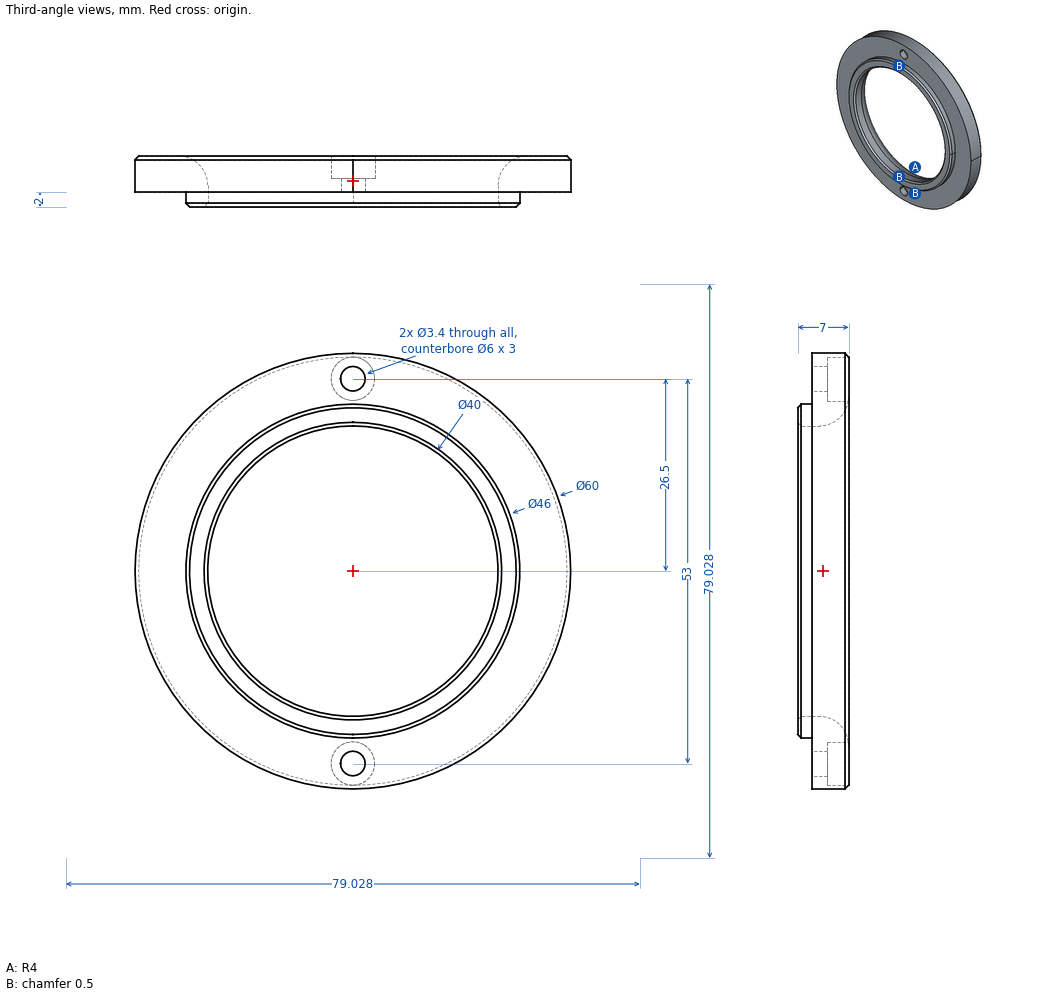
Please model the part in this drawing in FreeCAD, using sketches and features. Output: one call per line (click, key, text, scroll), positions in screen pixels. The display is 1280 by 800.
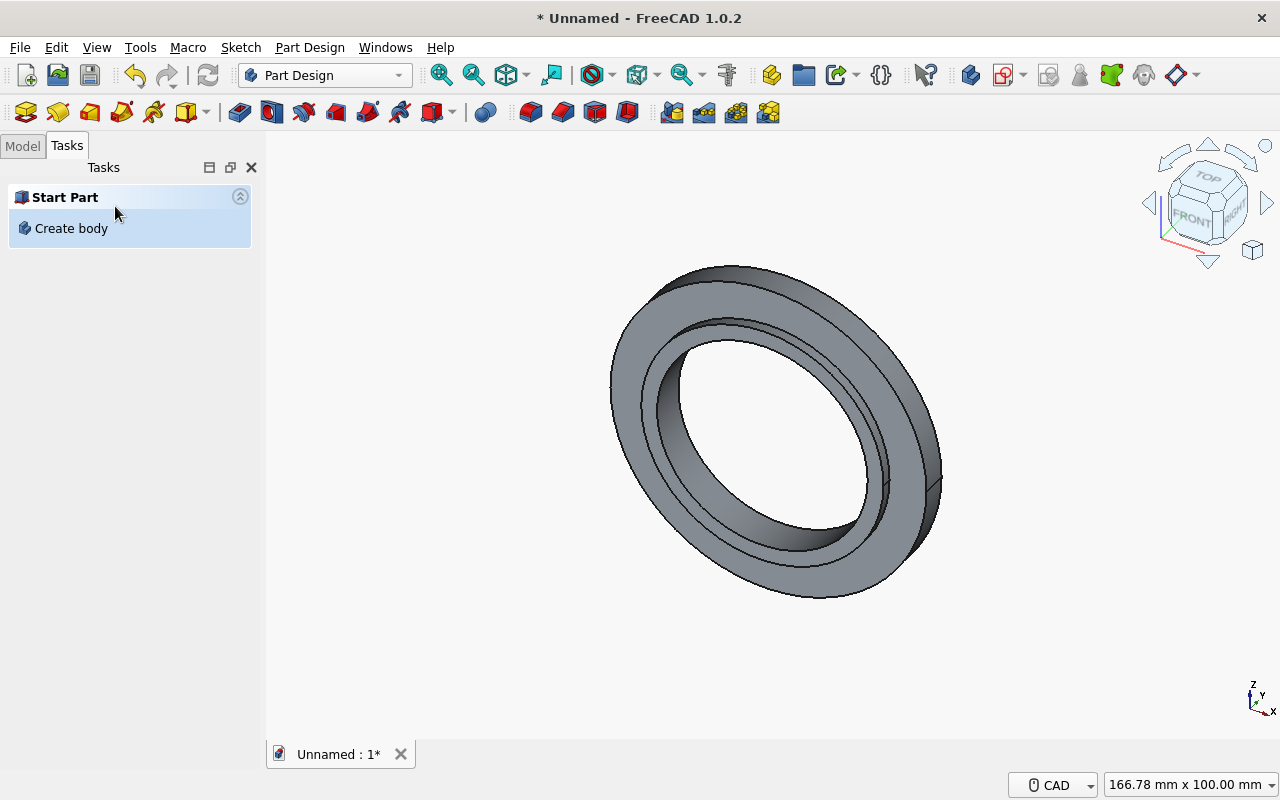
key(0)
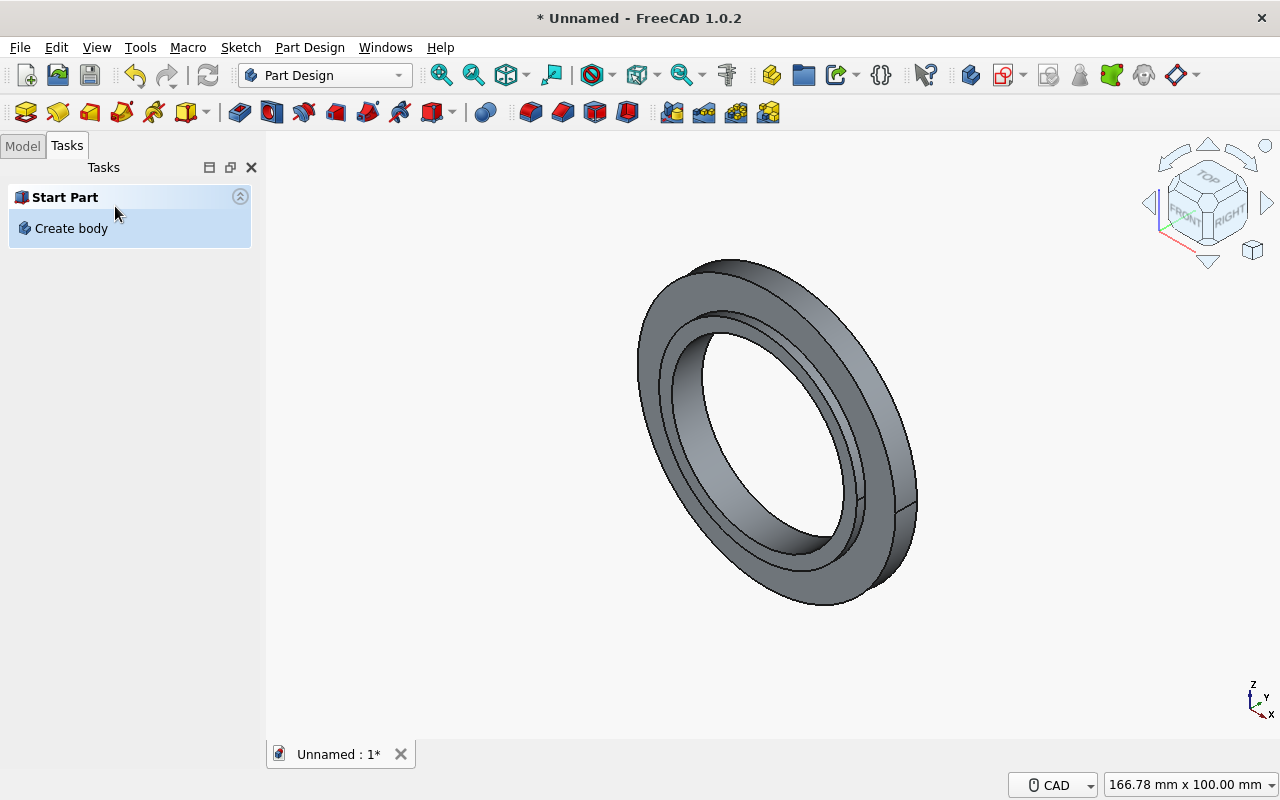
key(2)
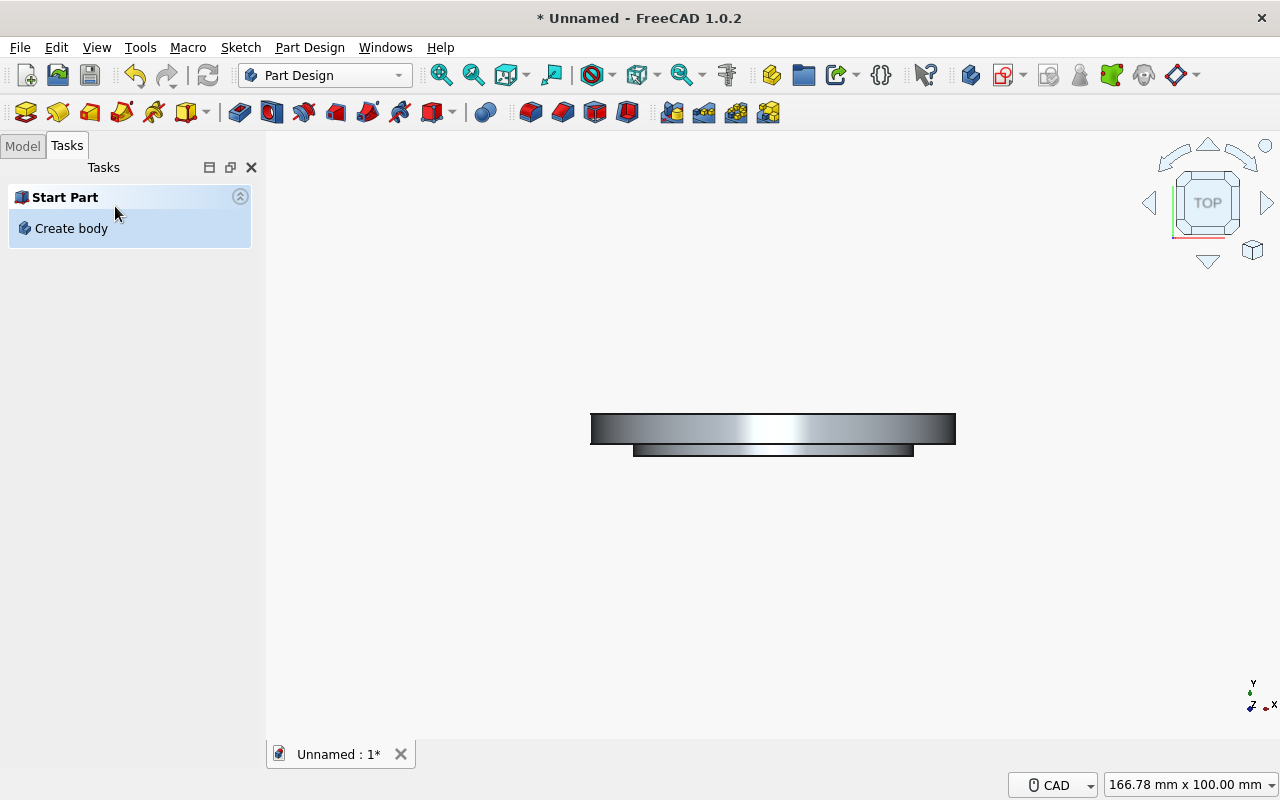
click(442, 76)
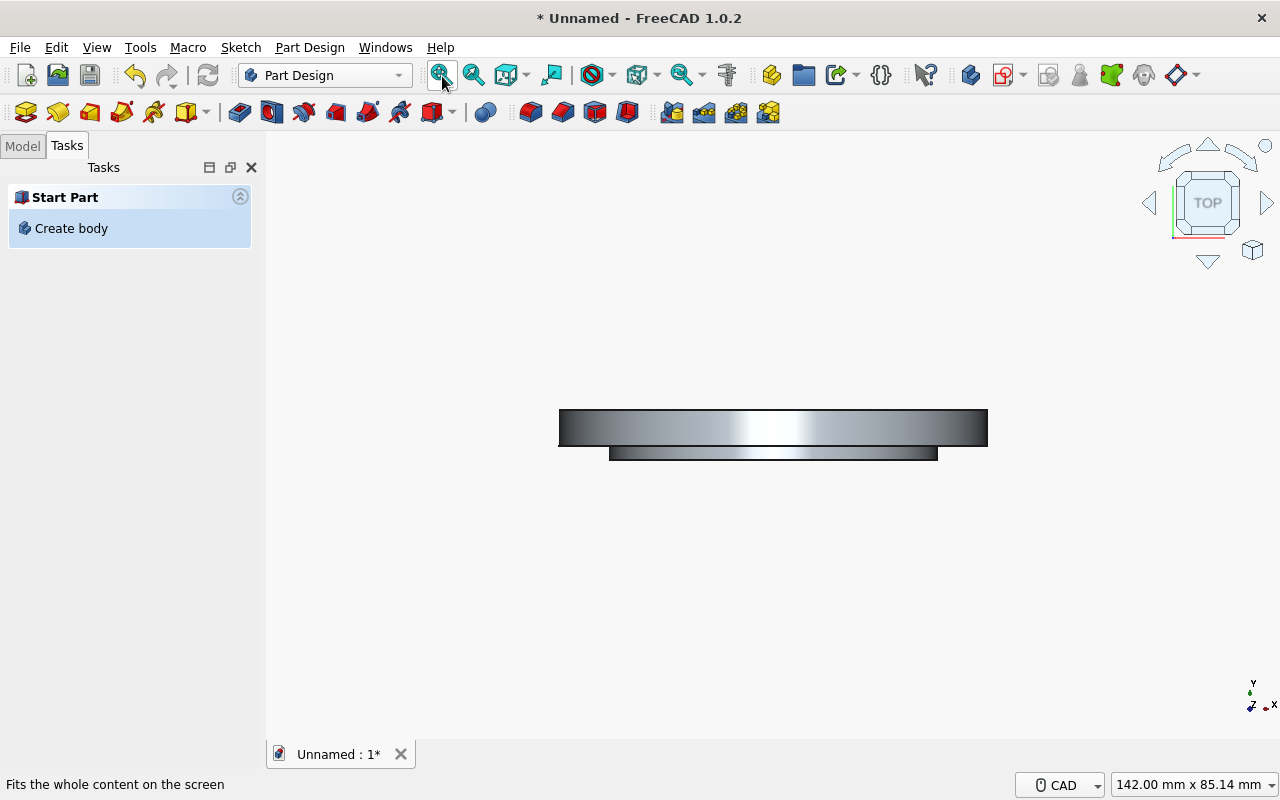
key(1)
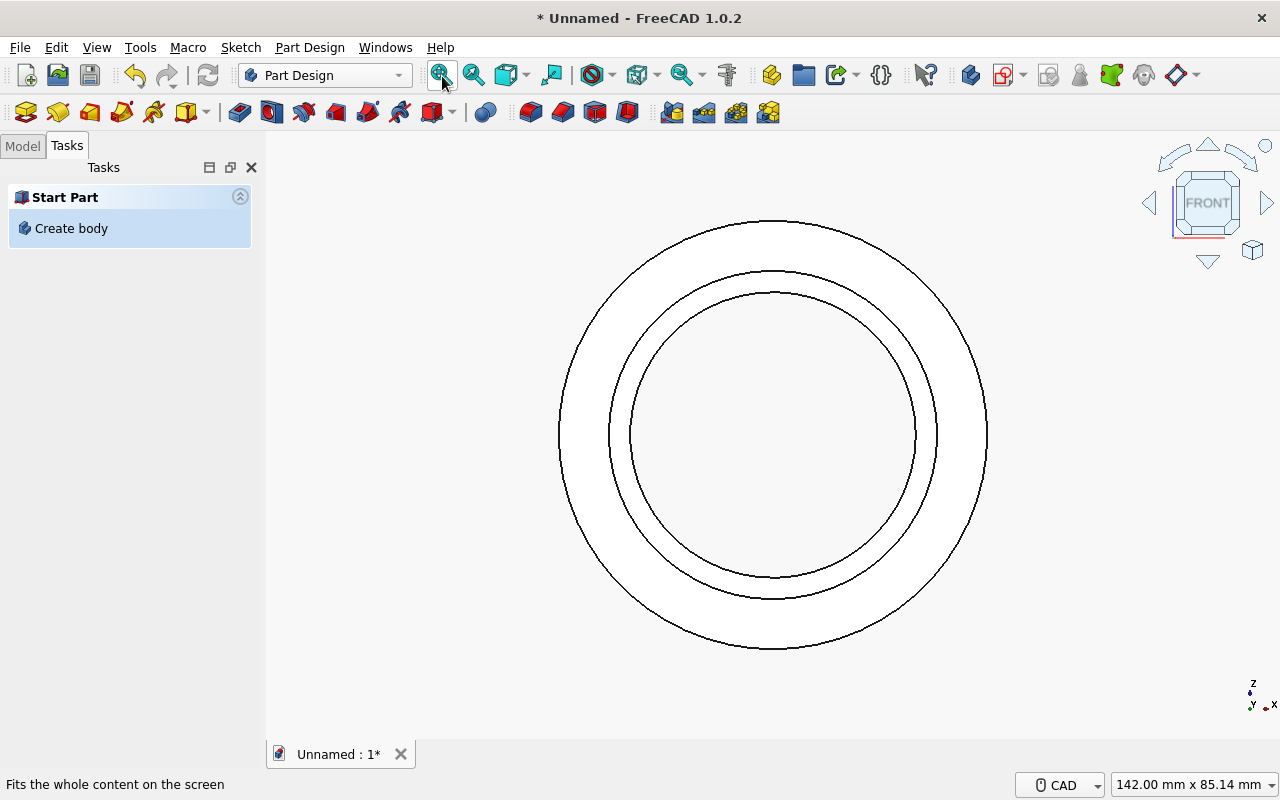
key(3)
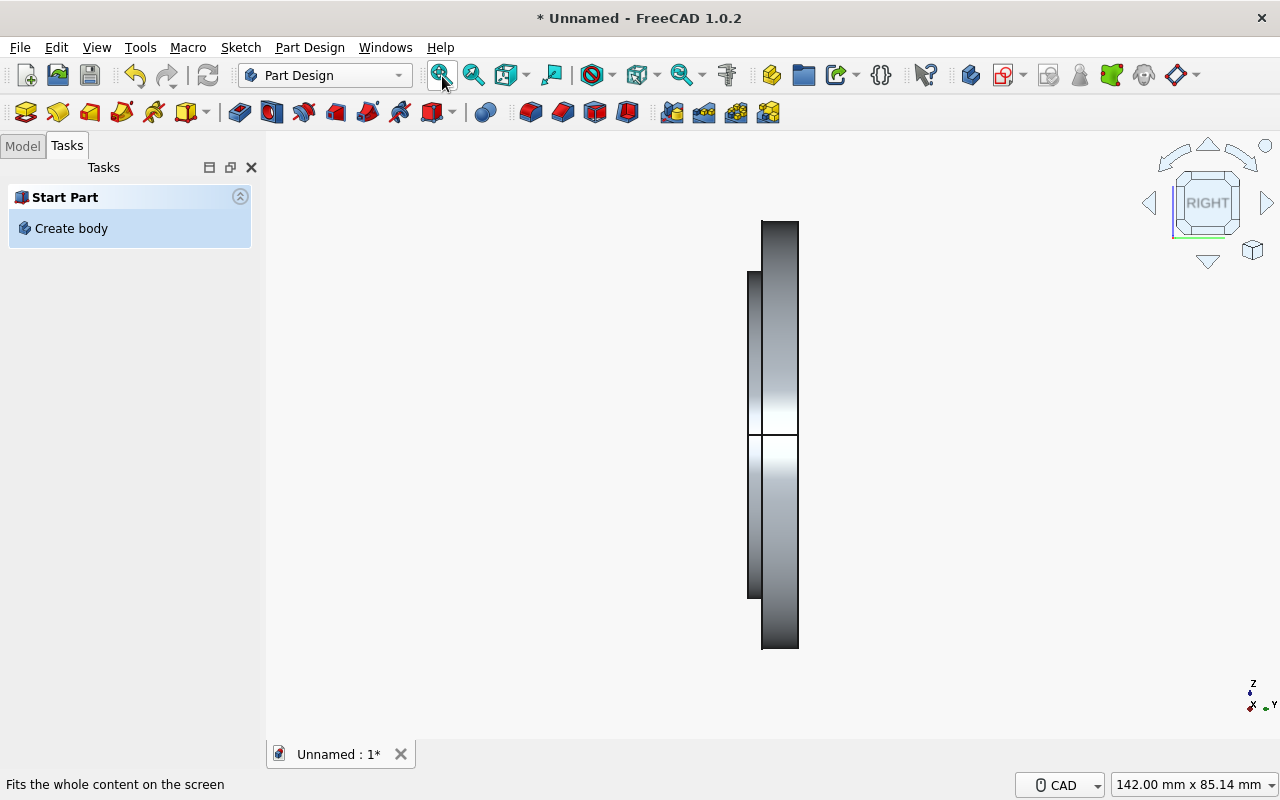
key(5)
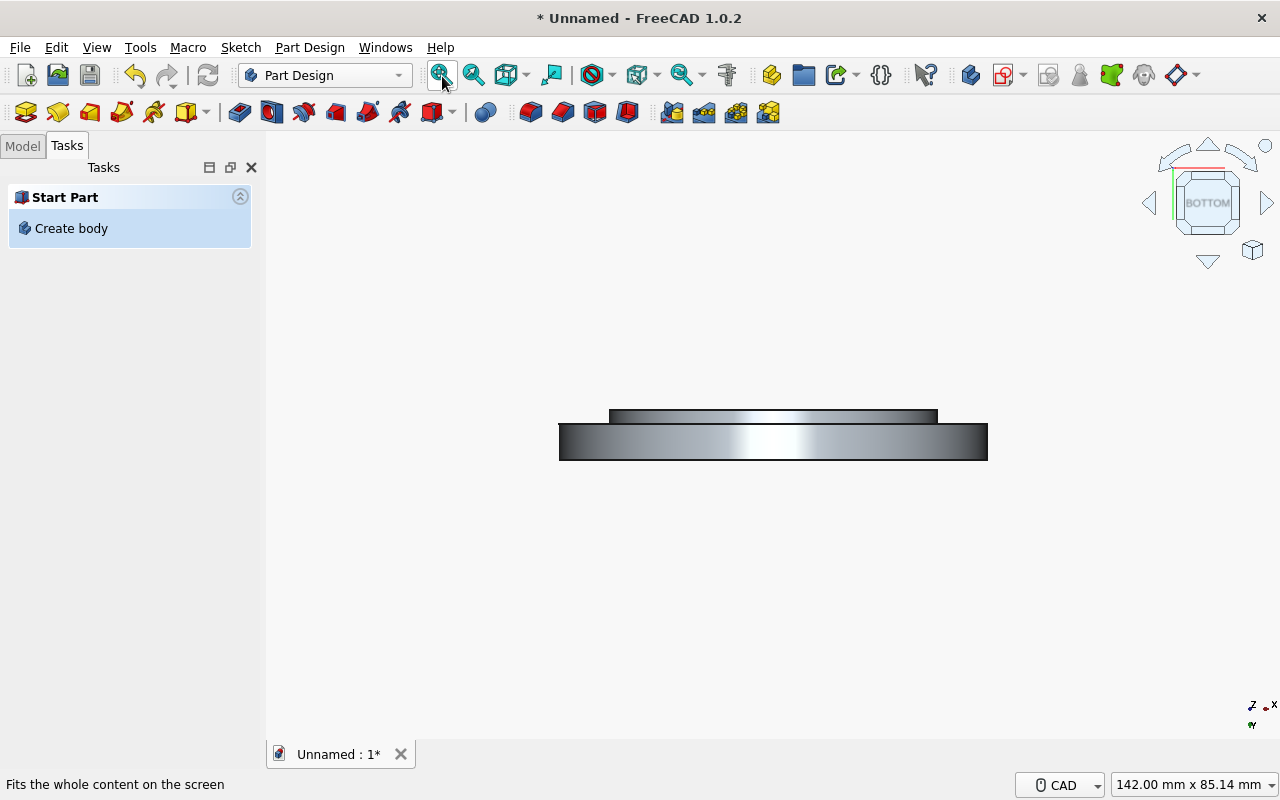
click(442, 76)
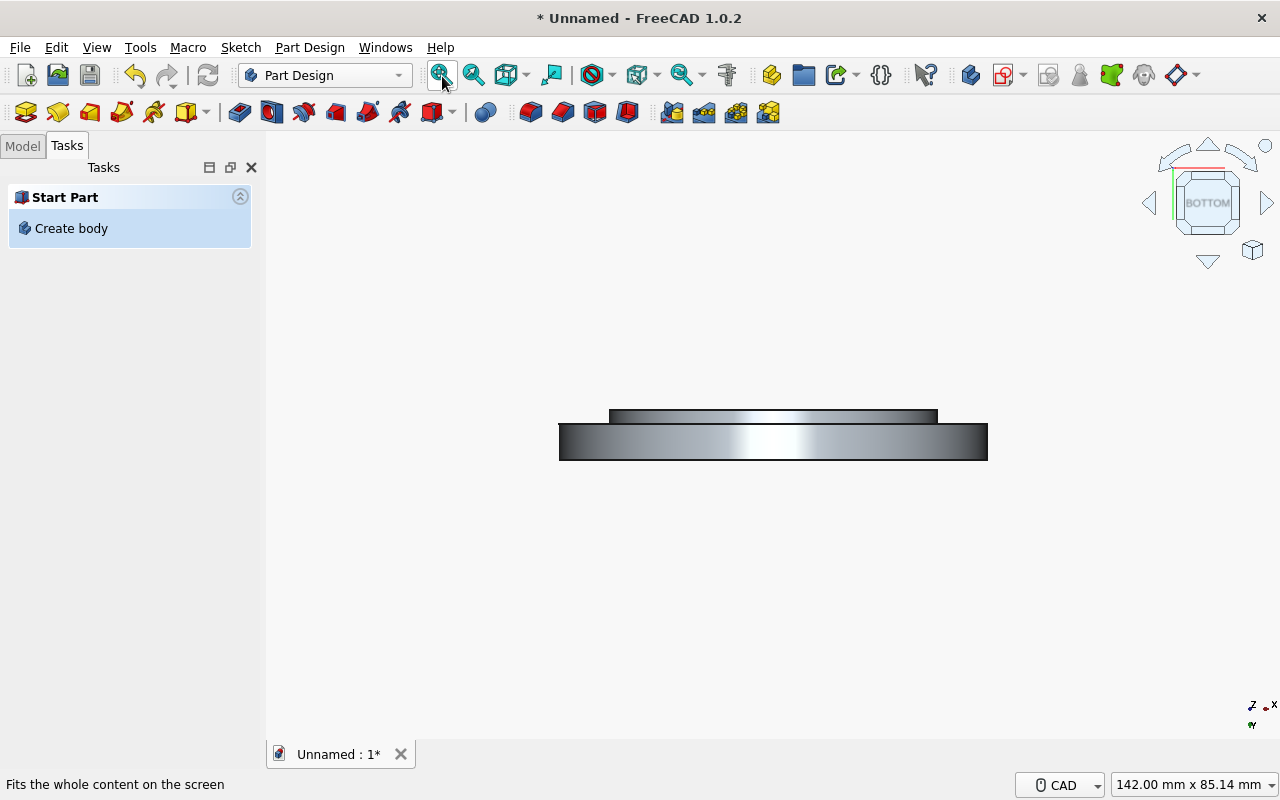
key(4)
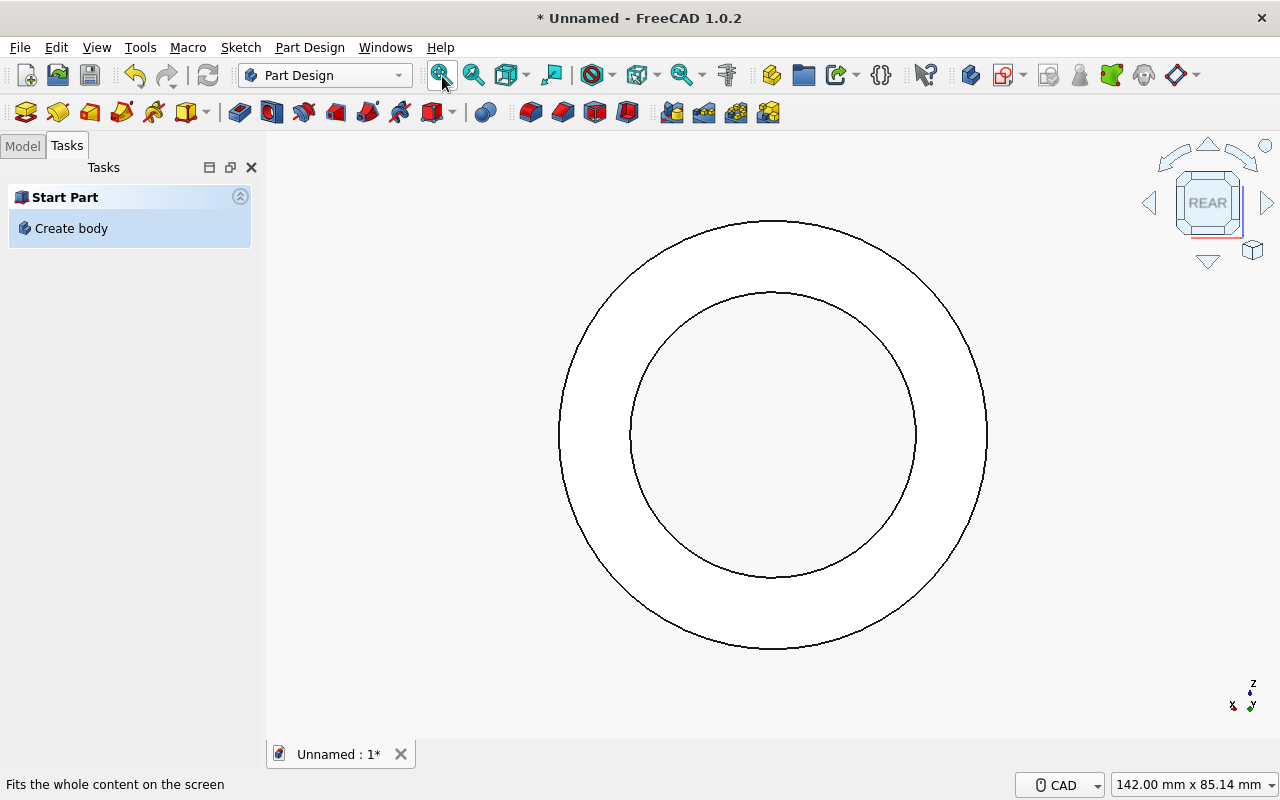
click(916, 434)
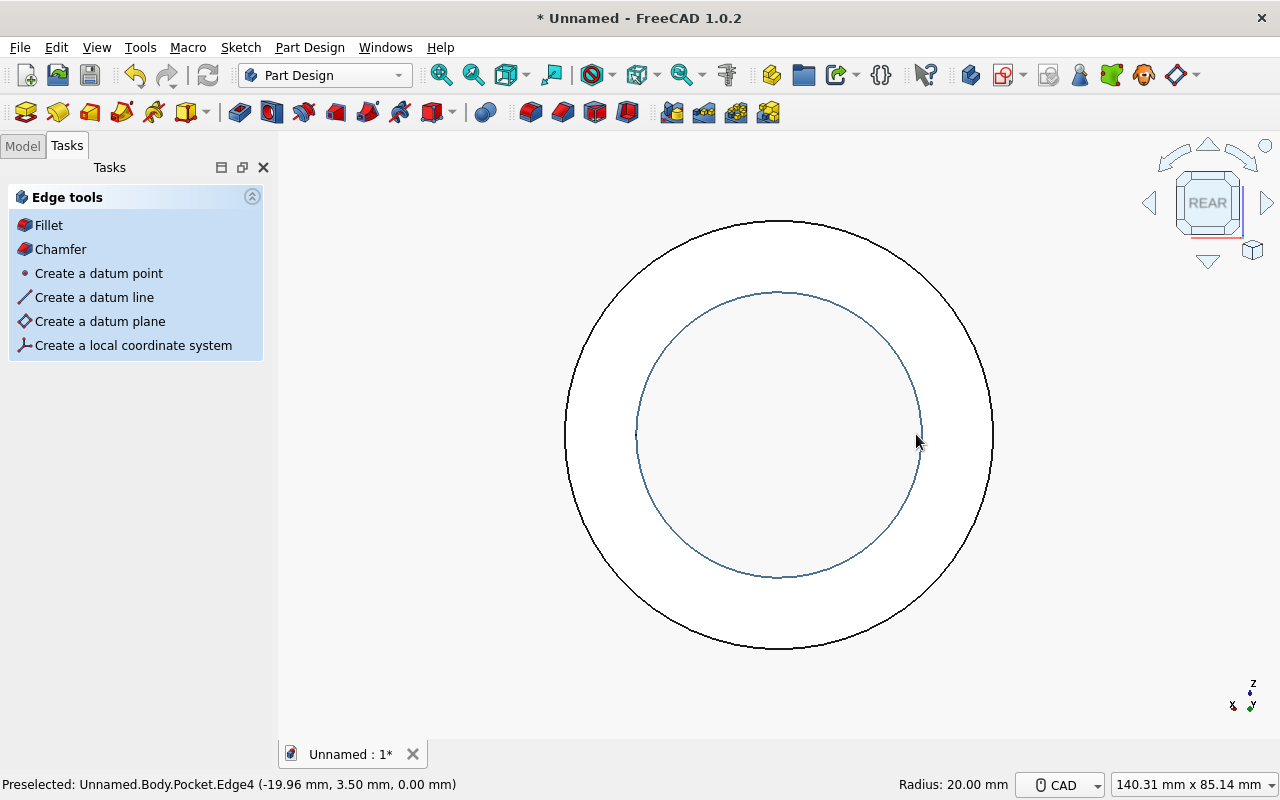
click(532, 112)